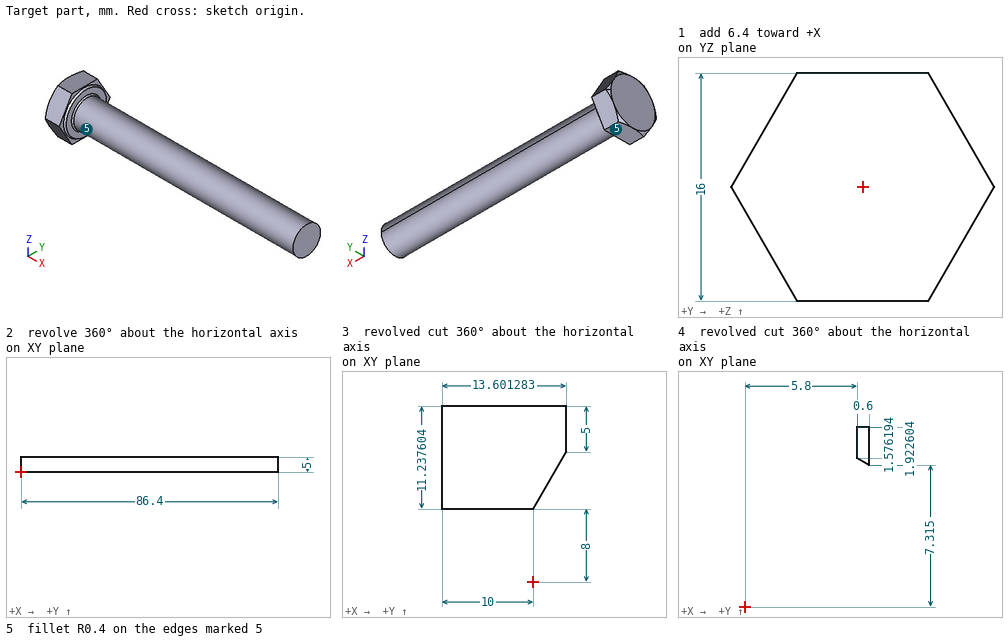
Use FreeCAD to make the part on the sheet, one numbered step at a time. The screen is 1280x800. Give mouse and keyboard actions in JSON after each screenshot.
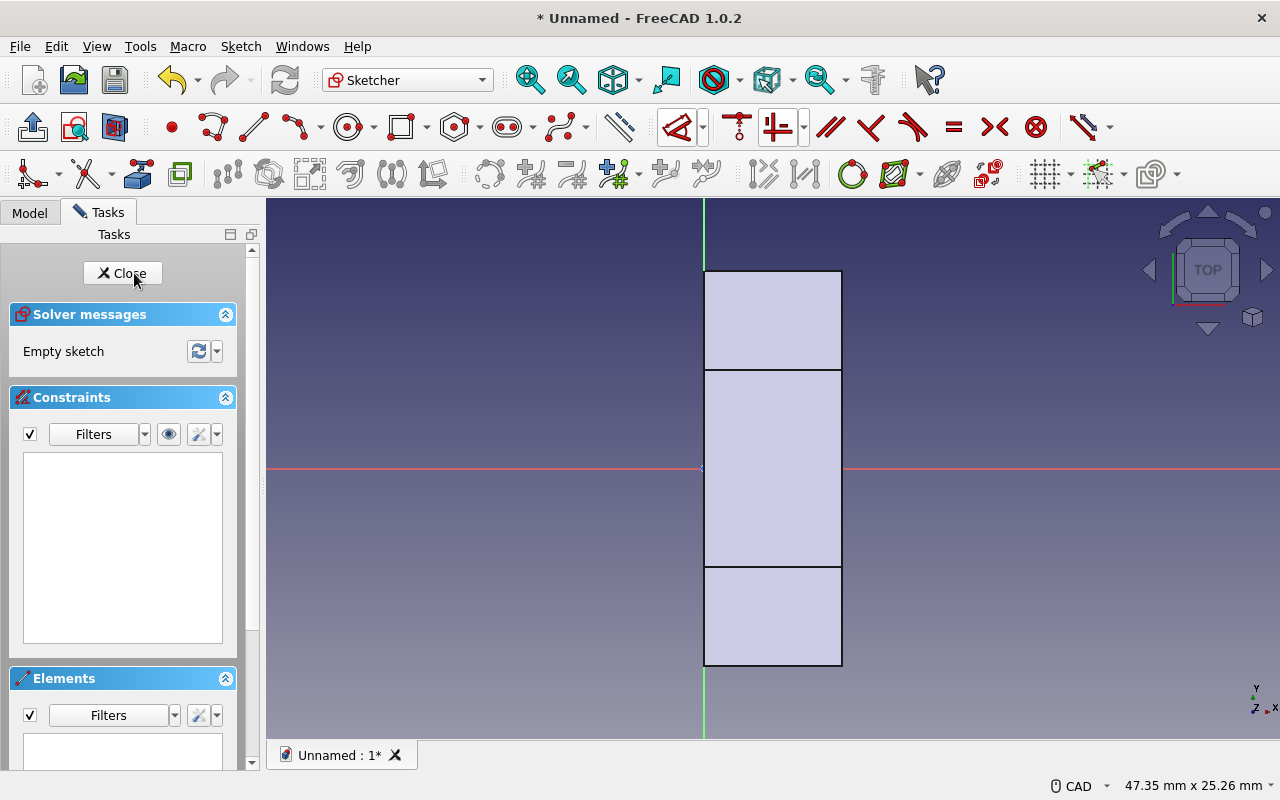
{"action": "left_click", "coordinate": [115, 128]}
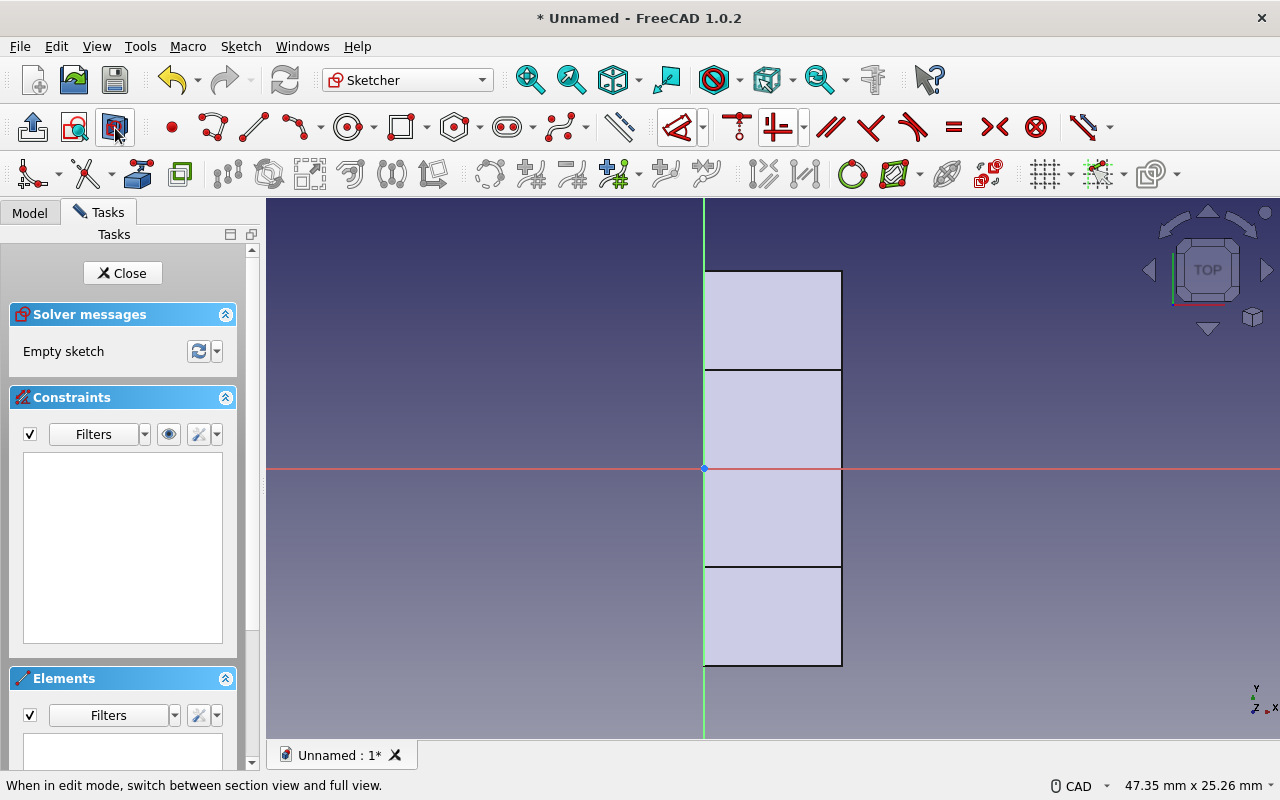
{"action": "scroll", "coordinate": [306, 492], "scroll_direction": "down", "scroll_amount": 6}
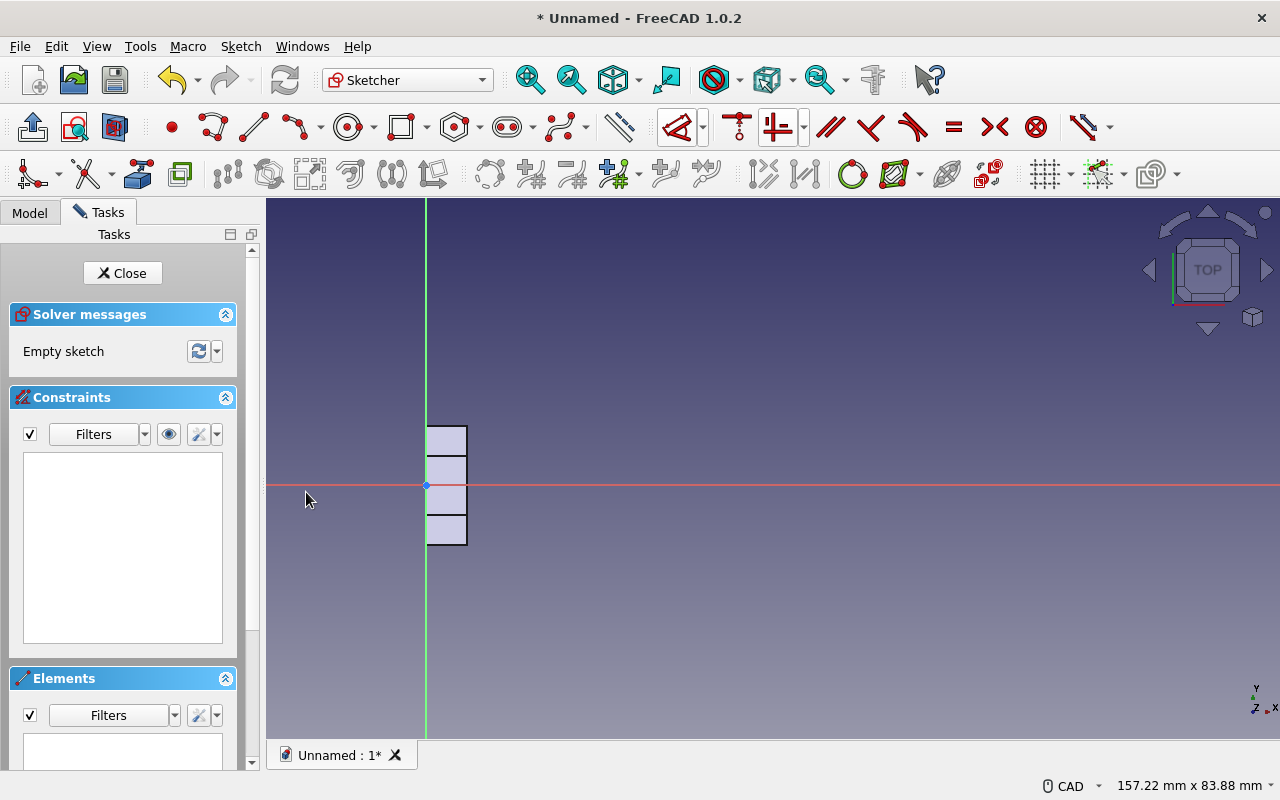
{"action": "left_click", "coordinate": [400, 128]}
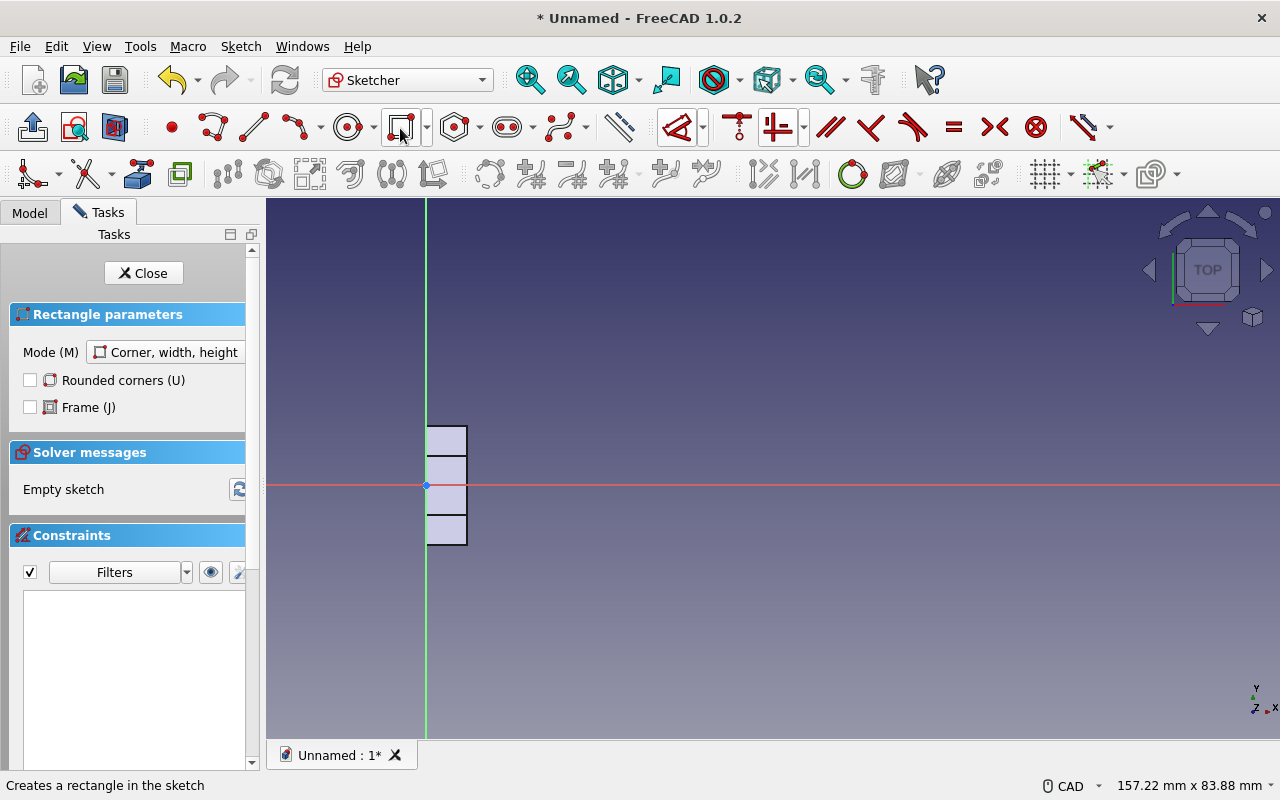
{"action": "left_click", "coordinate": [426, 485]}
{"action": "mouse_move", "coordinate": [983, 453]}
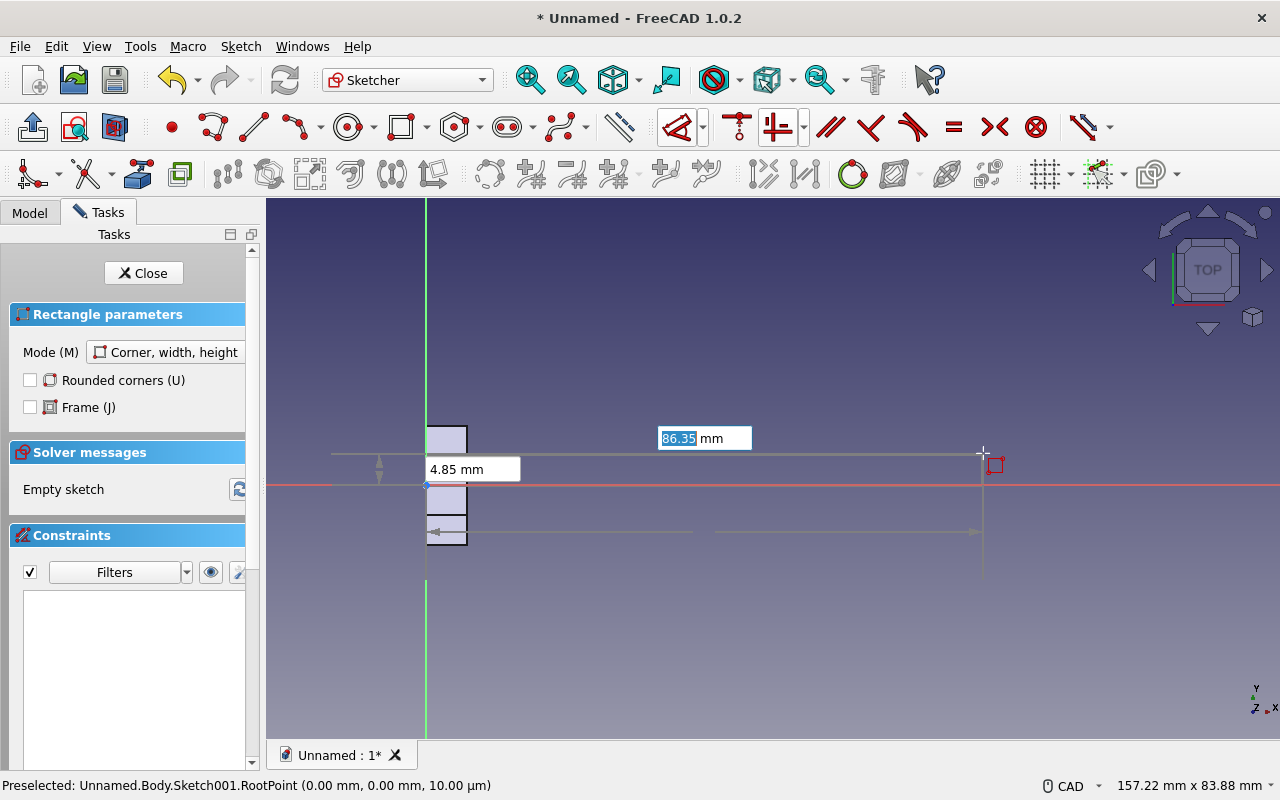
{"action": "type", "text": "86.4"}
{"action": "key", "text": "Tab"}
{"action": "type", "text": "5"}
{"action": "key", "text": "Return"}
{"action": "key", "text": "Escape"}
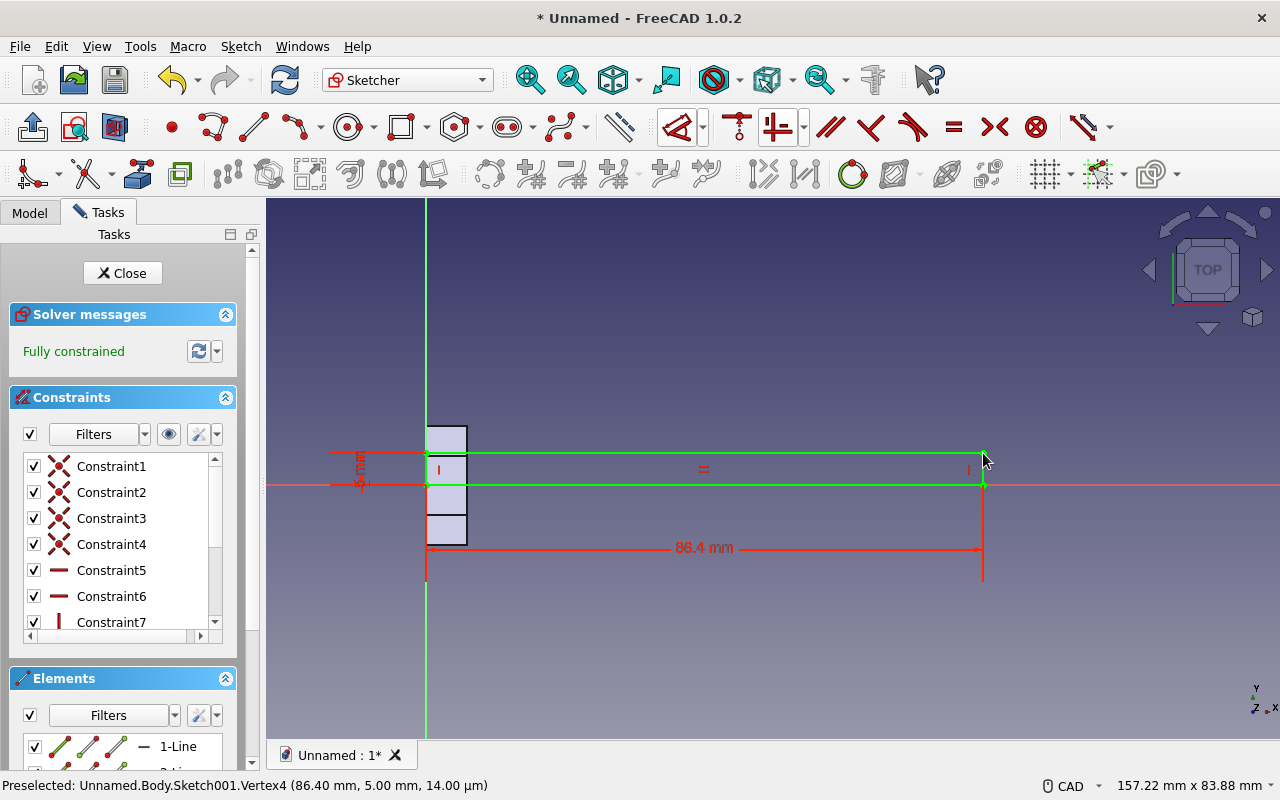
{"action": "left_click", "coordinate": [123, 273]}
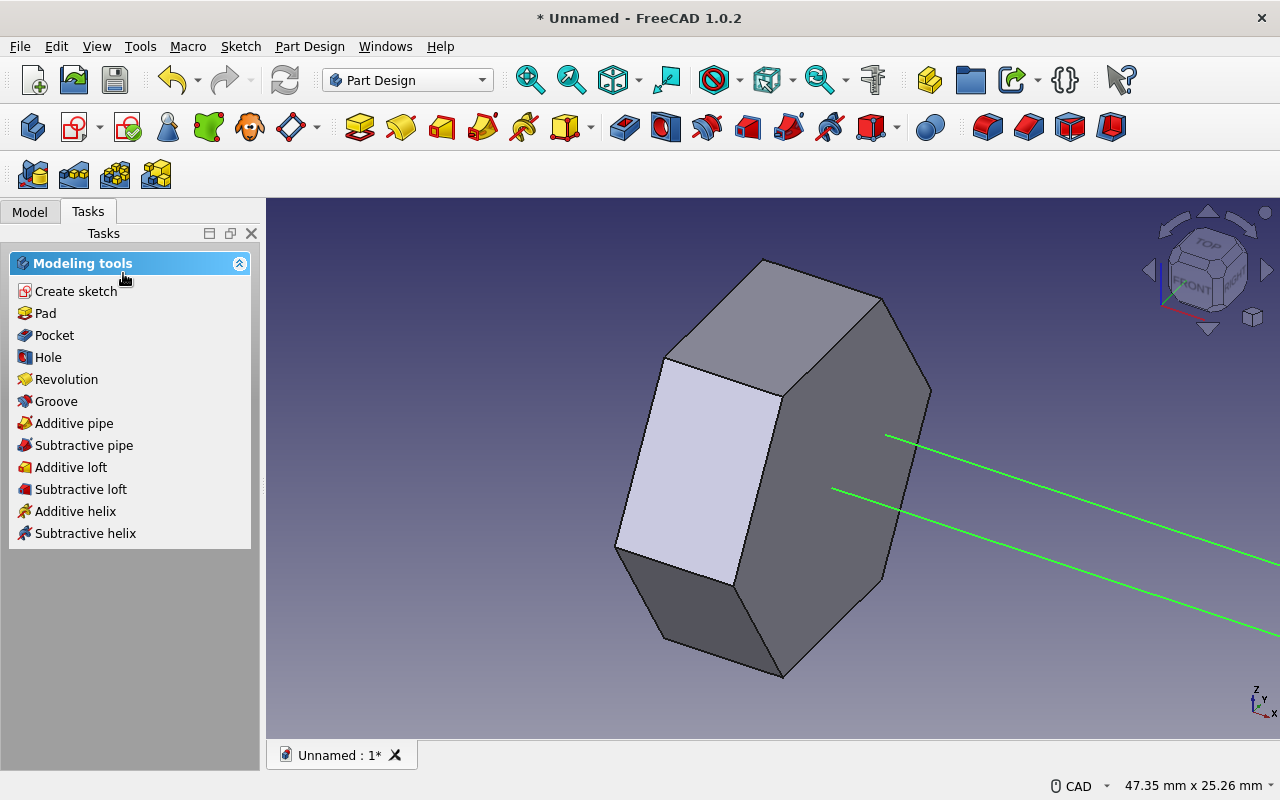
{"action": "left_click", "coordinate": [401, 128]}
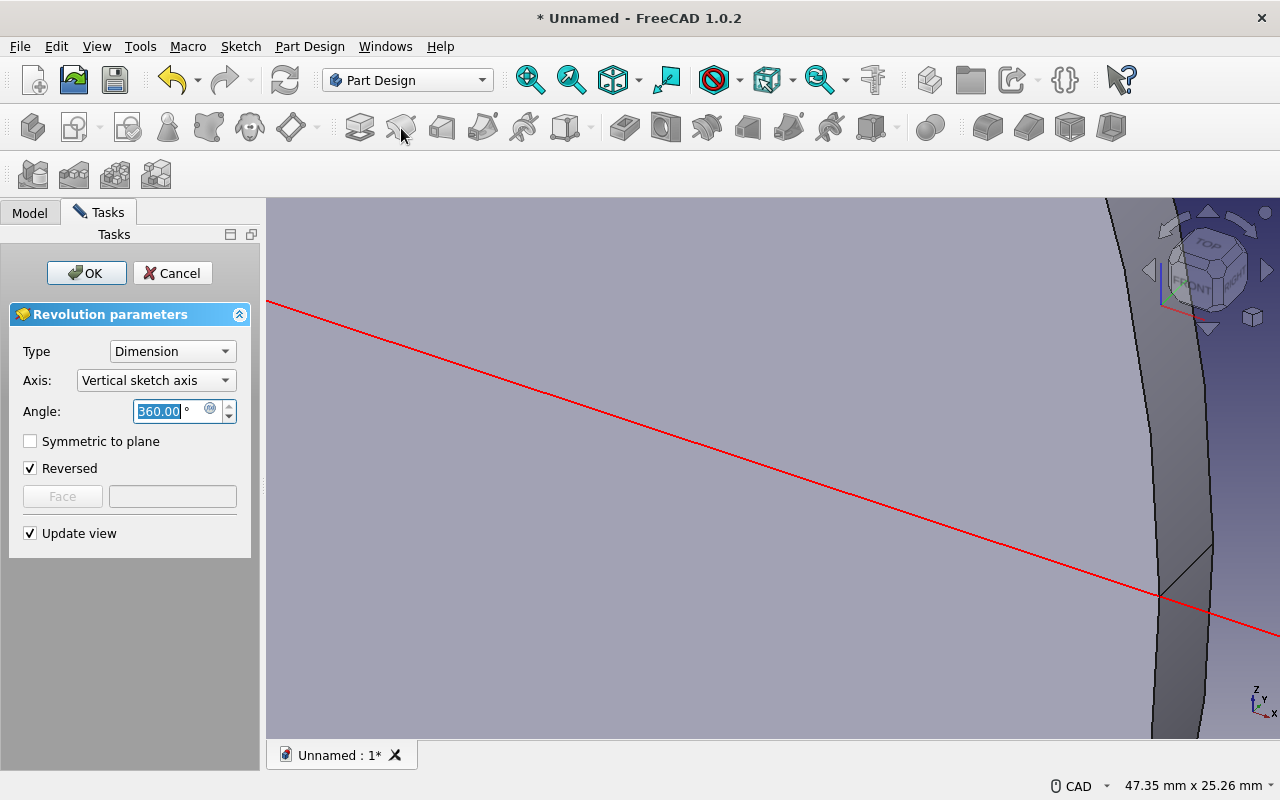
{"action": "left_click", "coordinate": [157, 380]}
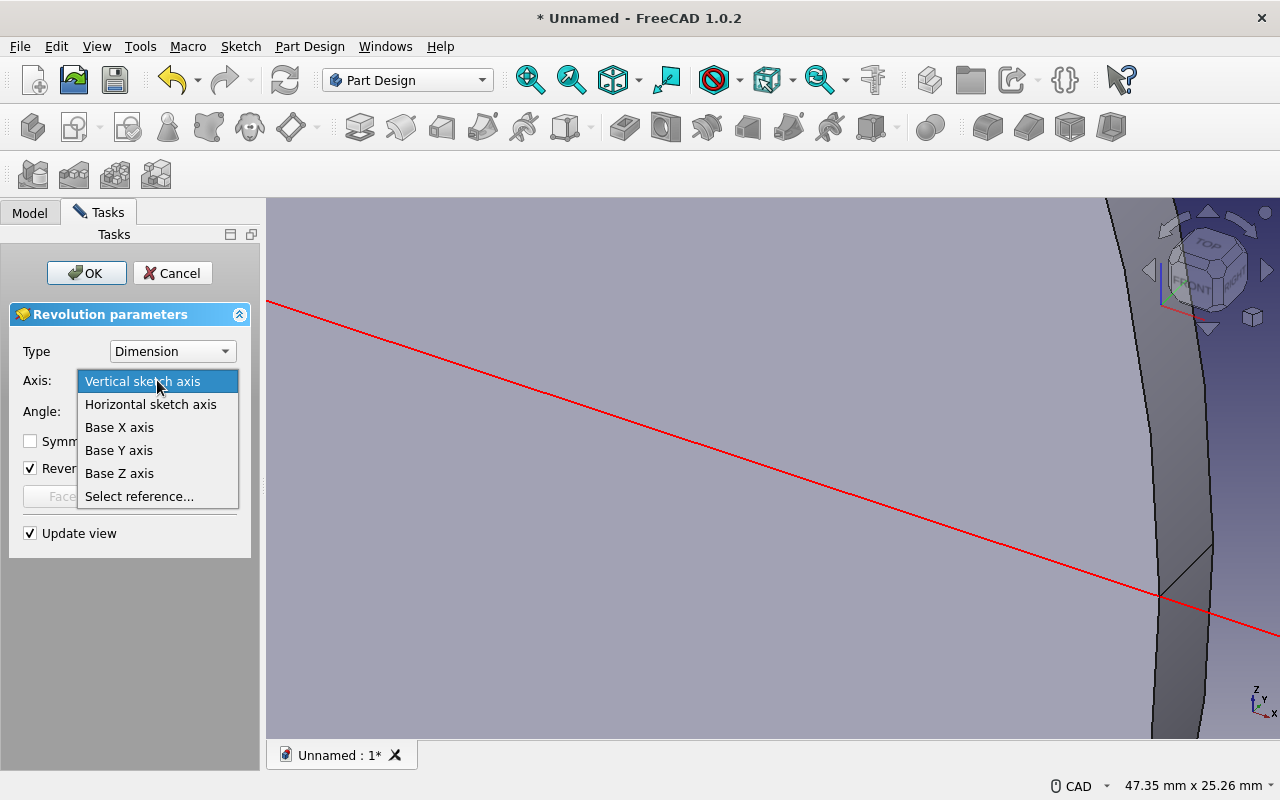
{"action": "left_click", "coordinate": [156, 404]}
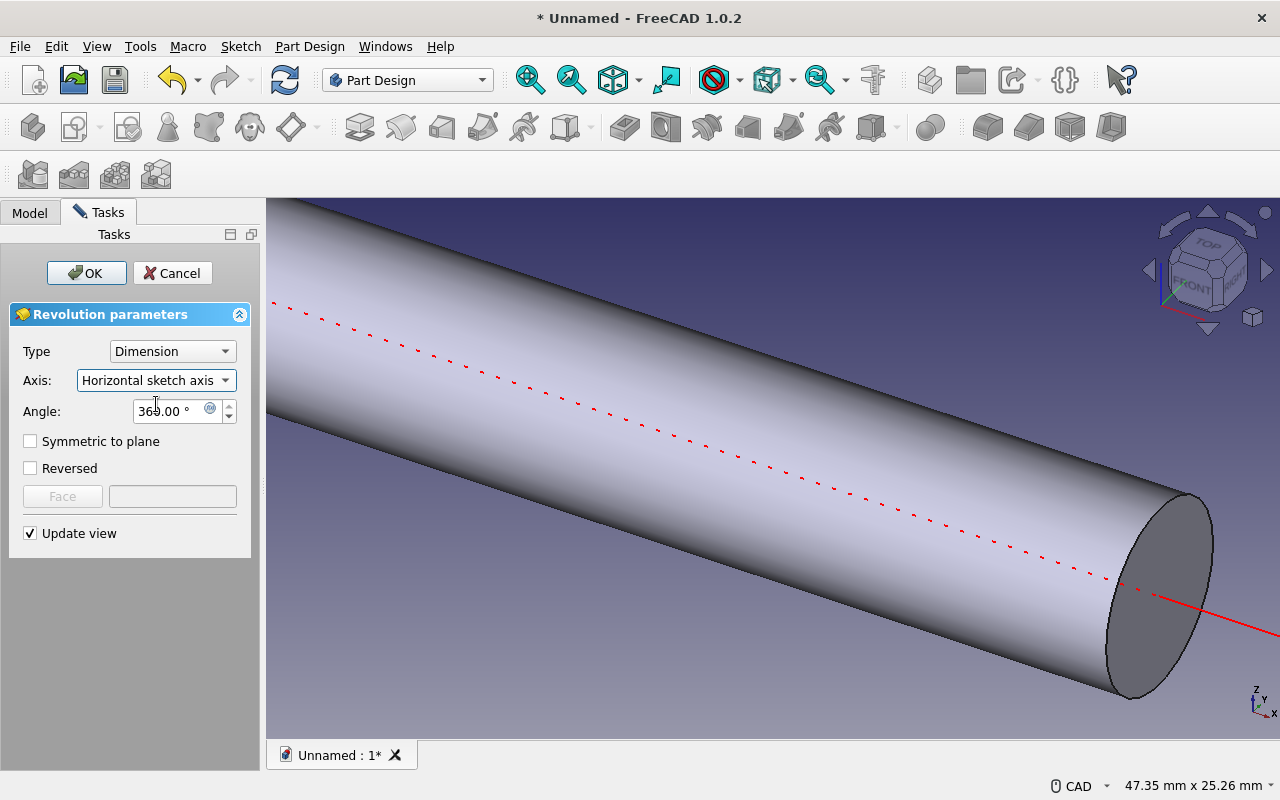
{"action": "left_click", "coordinate": [87, 273]}